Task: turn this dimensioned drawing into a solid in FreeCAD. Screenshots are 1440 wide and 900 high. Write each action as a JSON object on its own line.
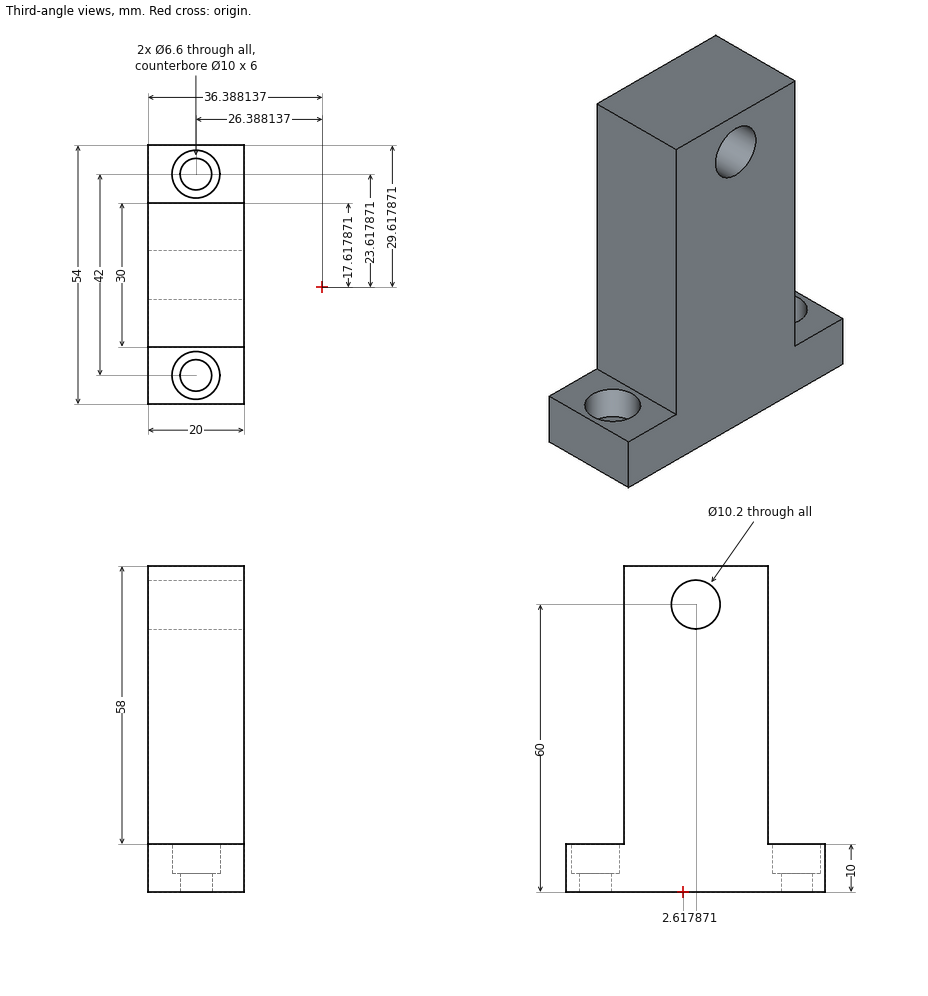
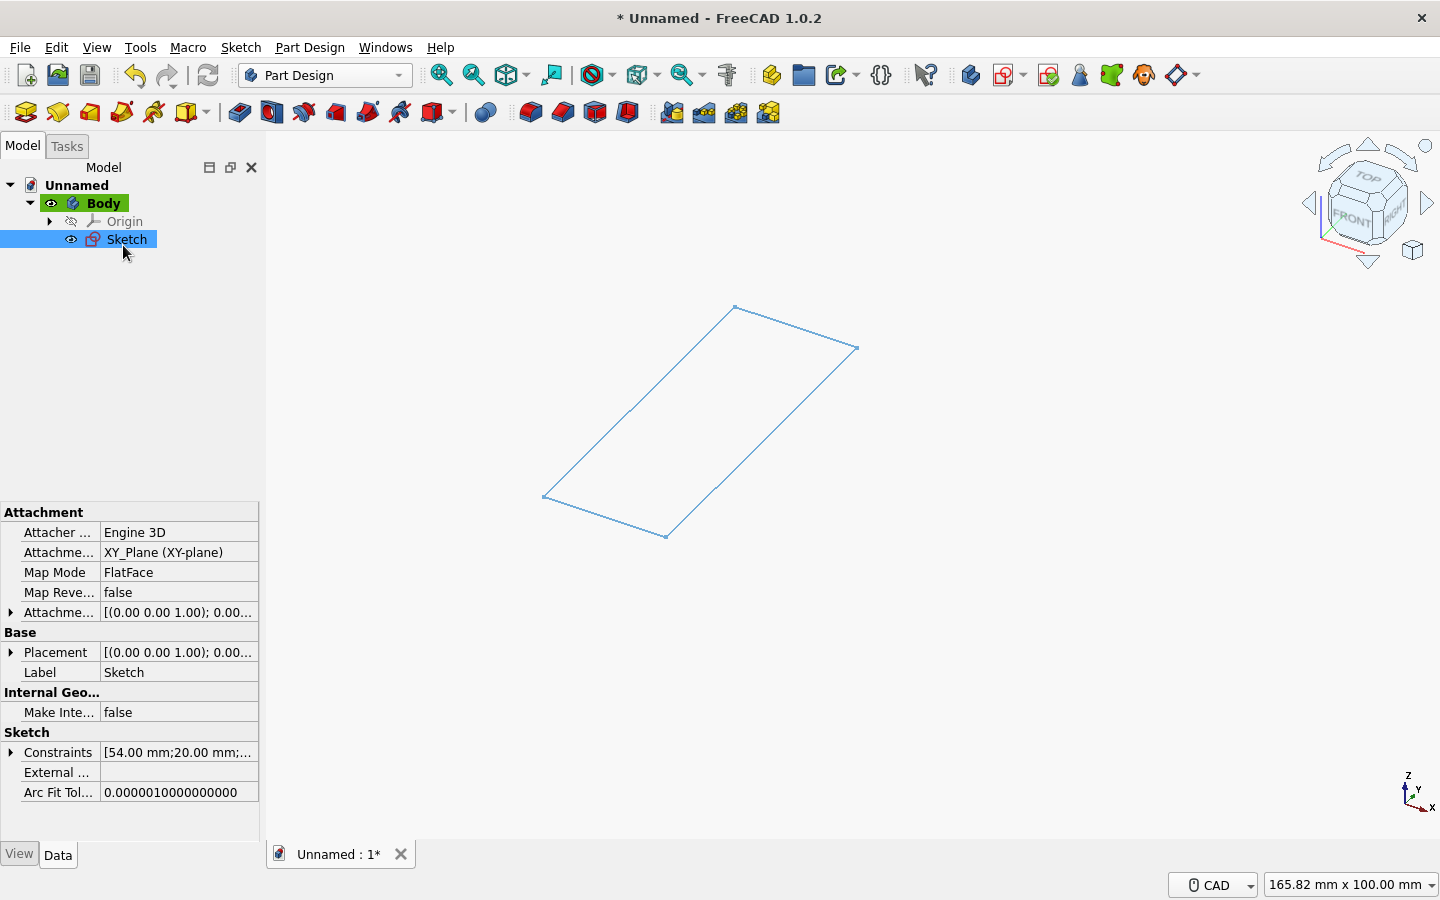
{"action": "left_click", "coordinate": [26, 112]}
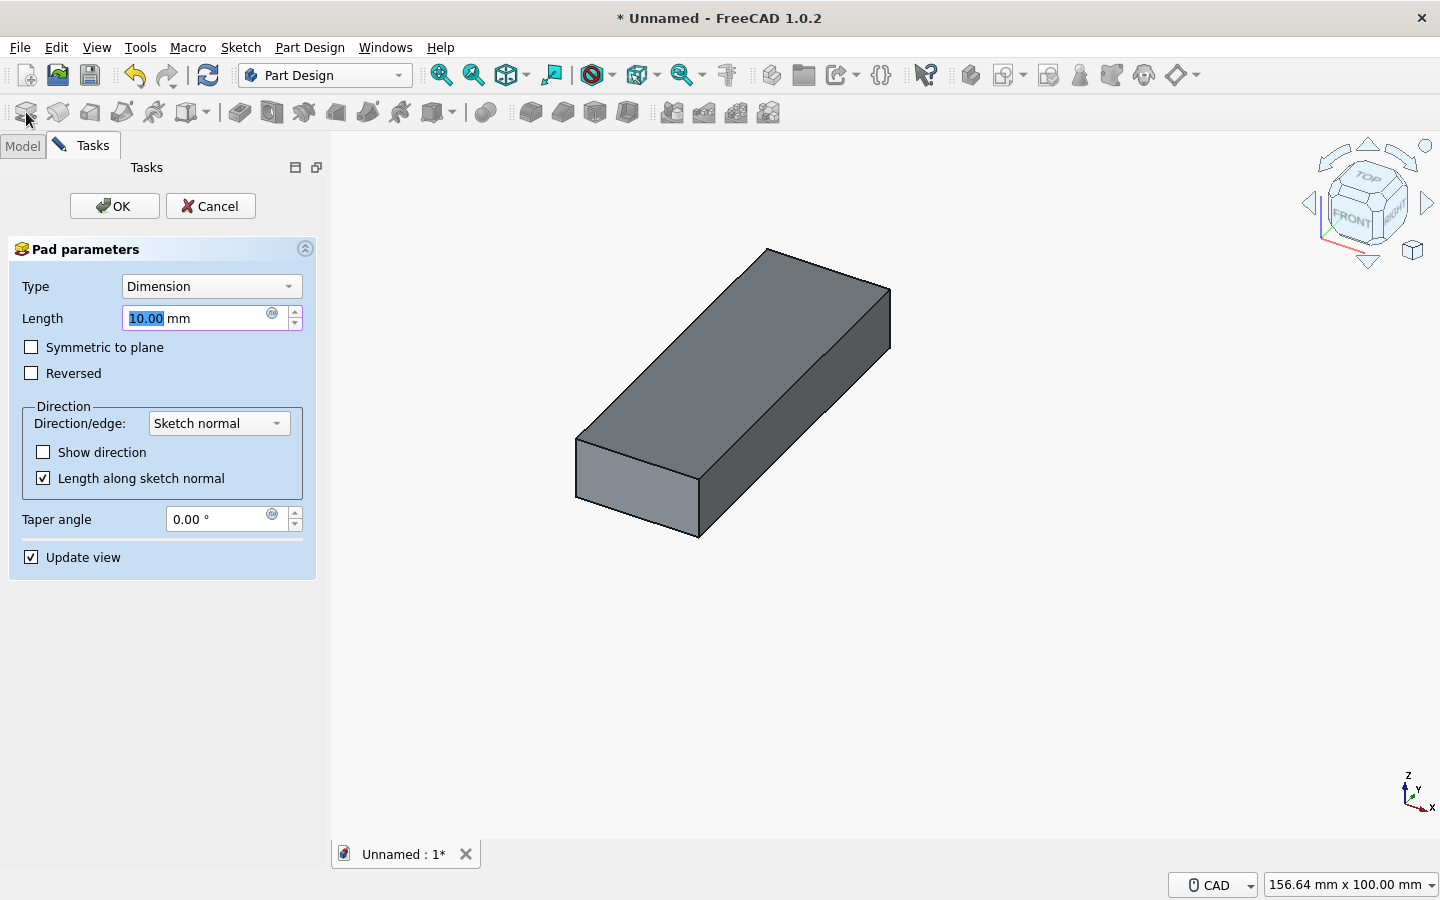
{"action": "type", "text": "10"}
{"action": "key", "text": "Tab"}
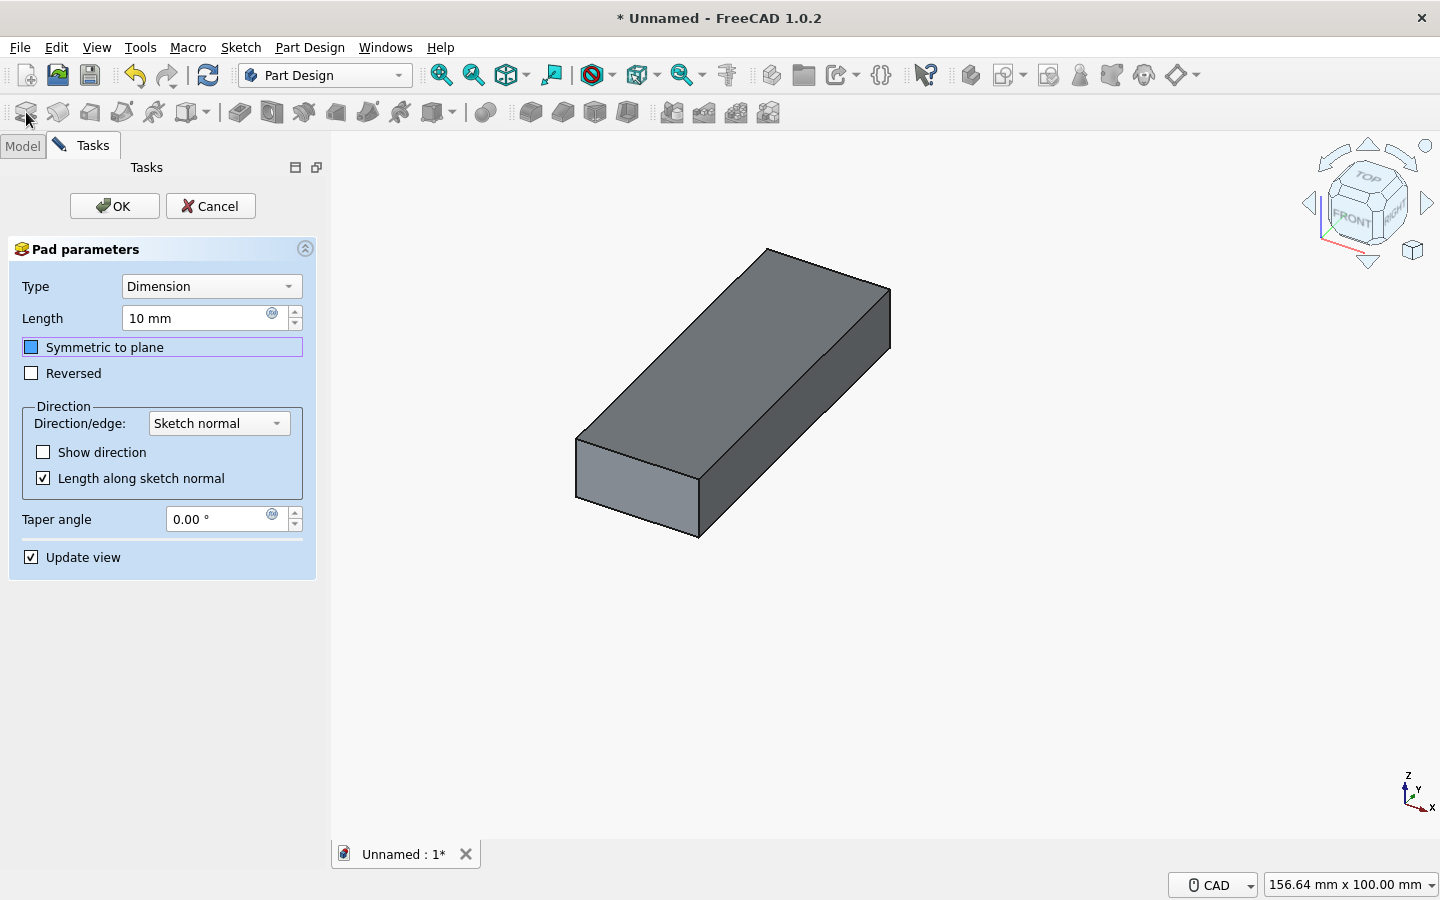
{"action": "left_click", "coordinate": [115, 206]}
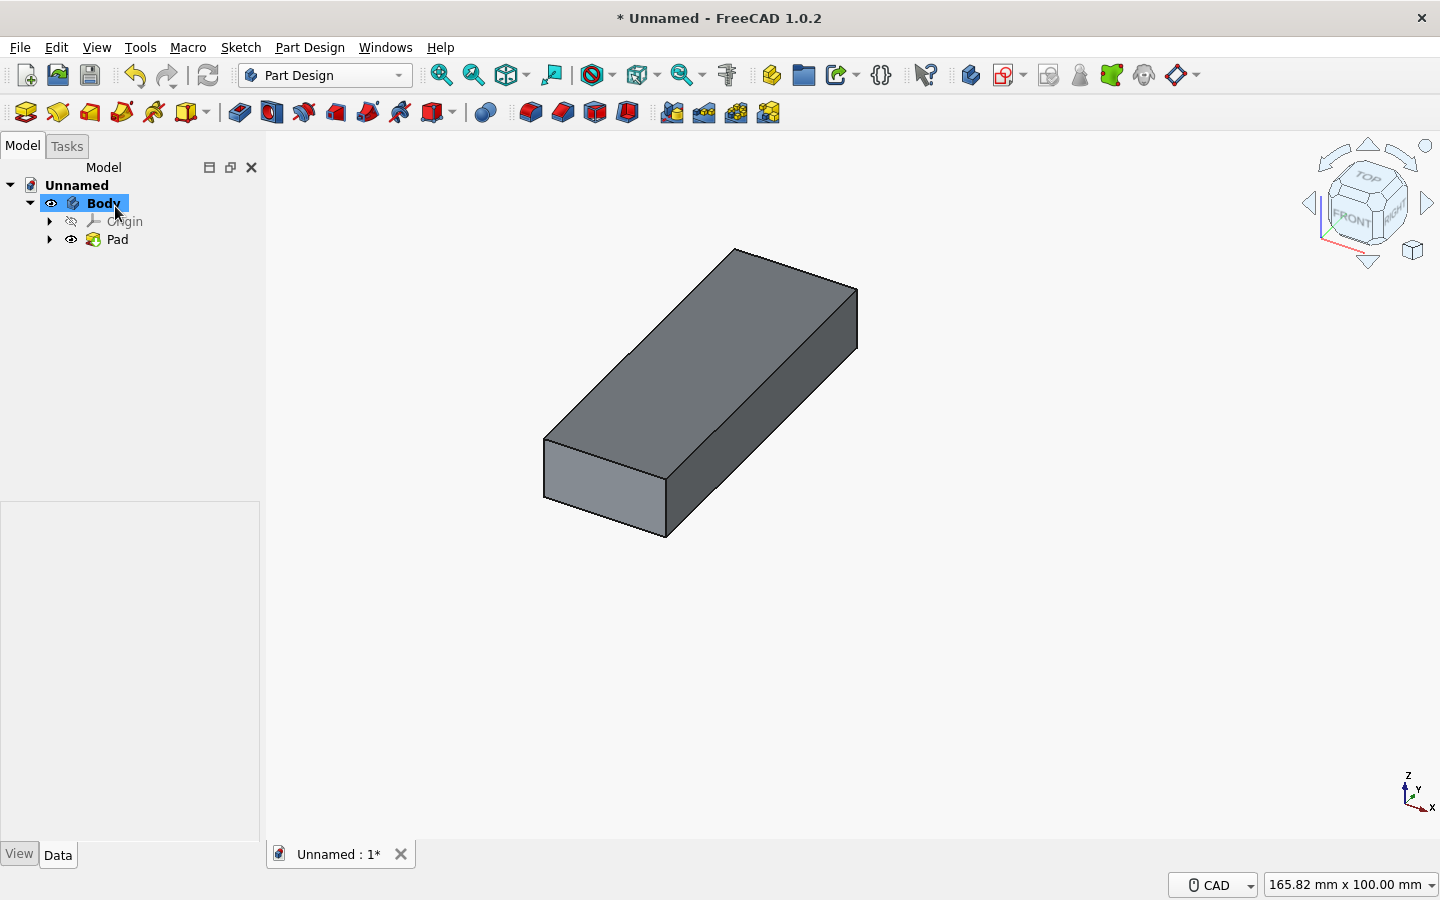
{"action": "left_click", "coordinate": [442, 76]}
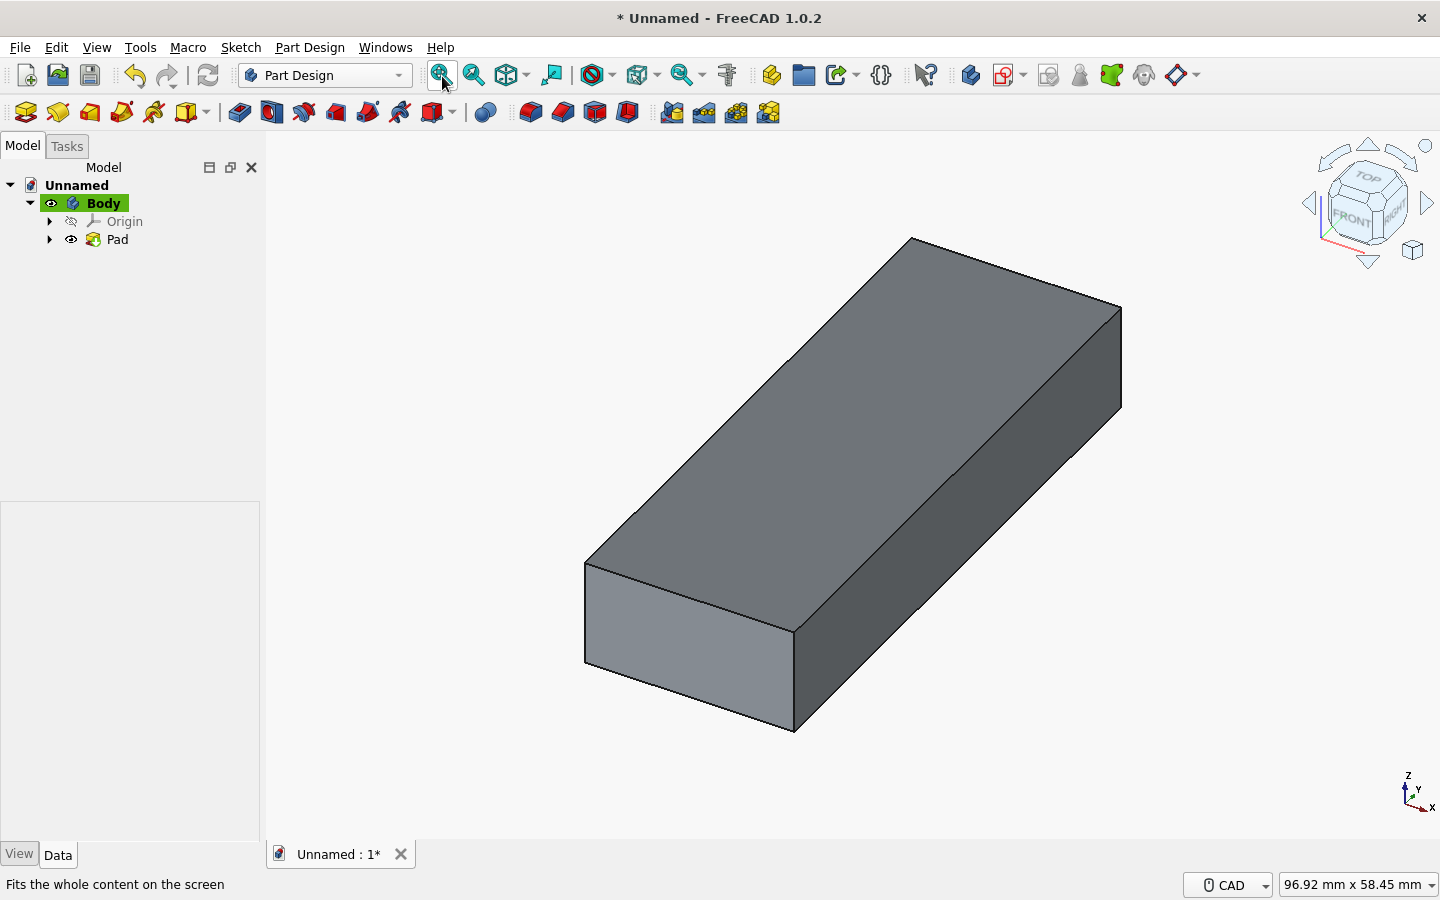
{"action": "left_click", "coordinate": [946, 342]}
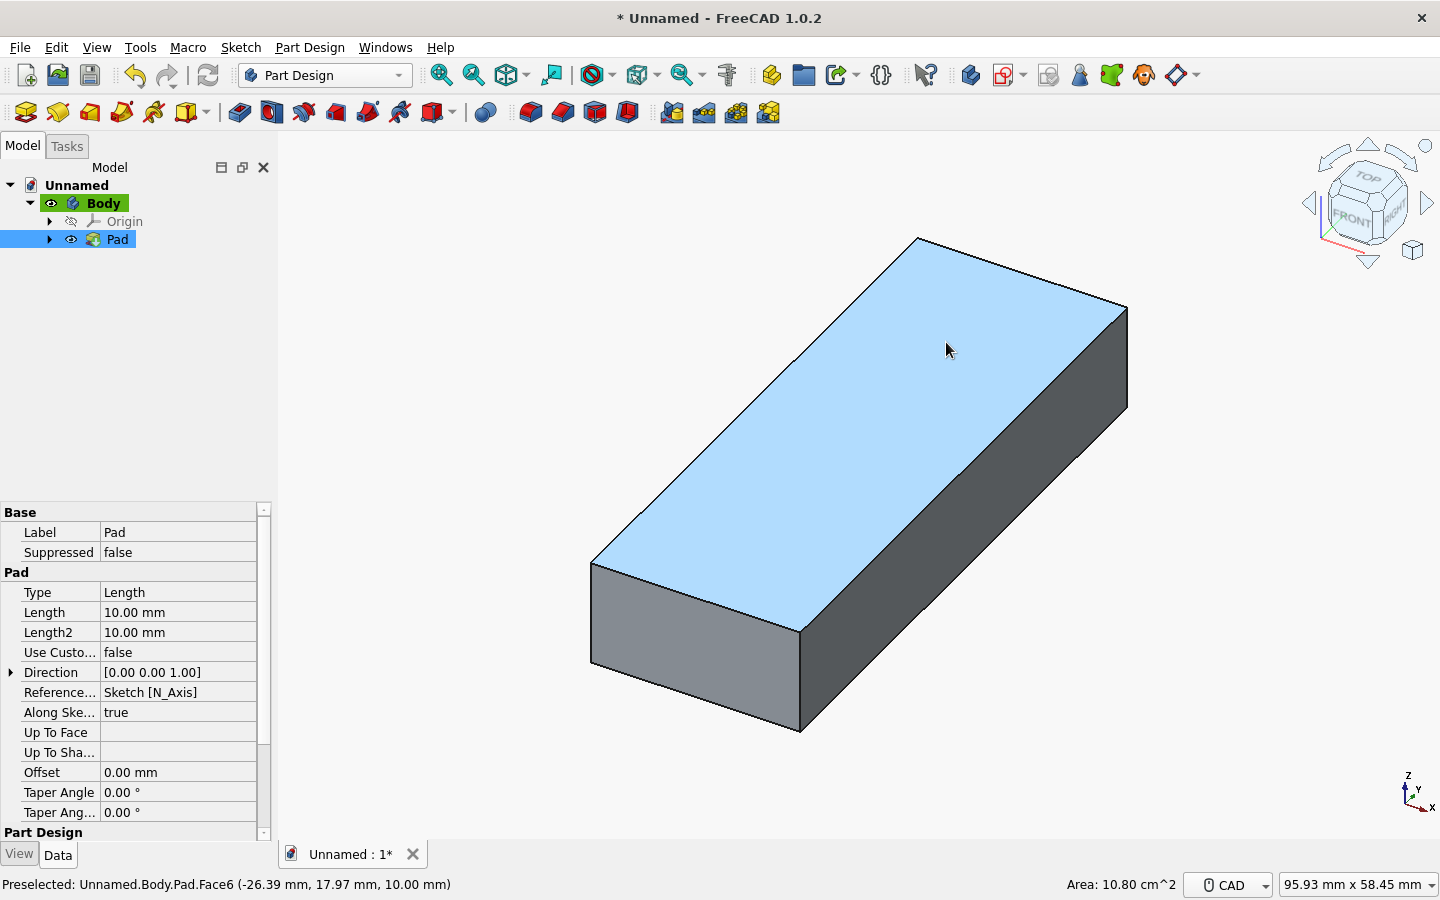
{"action": "left_click", "coordinate": [1004, 76]}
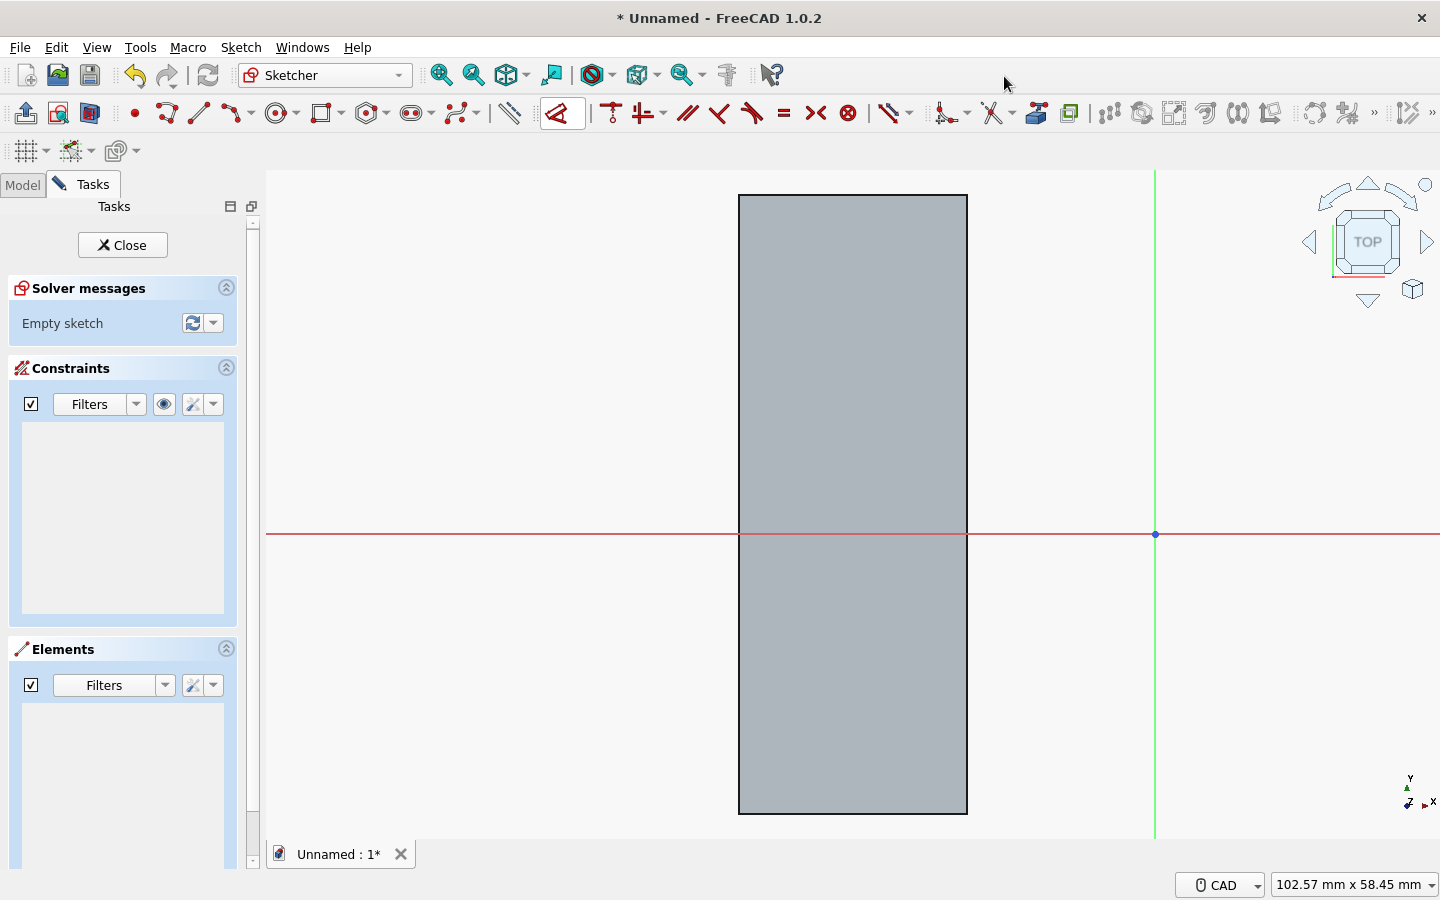
{"action": "left_click", "coordinate": [322, 114]}